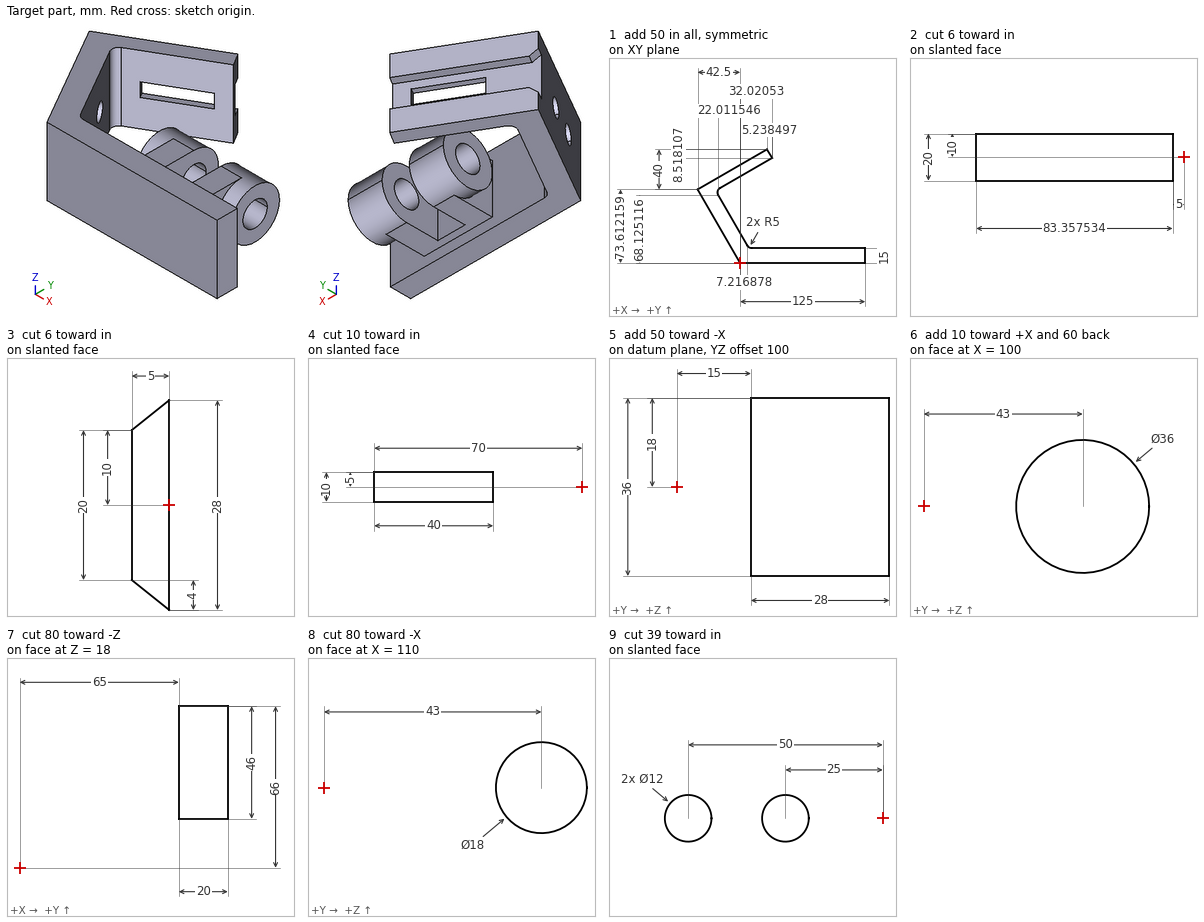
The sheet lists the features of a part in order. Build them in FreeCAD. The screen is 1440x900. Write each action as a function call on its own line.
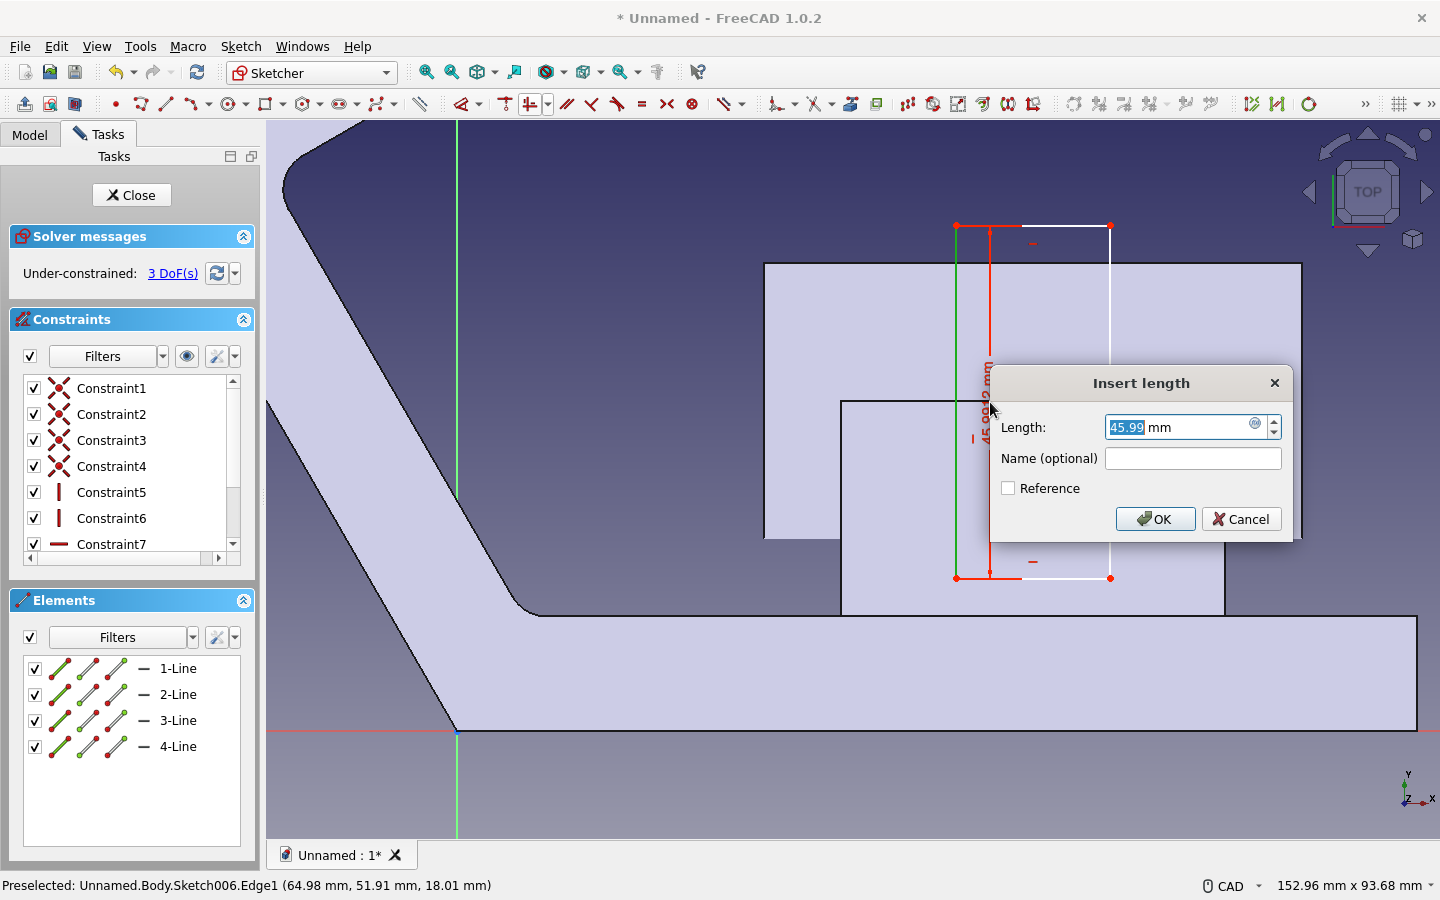
text(46)
key(Return)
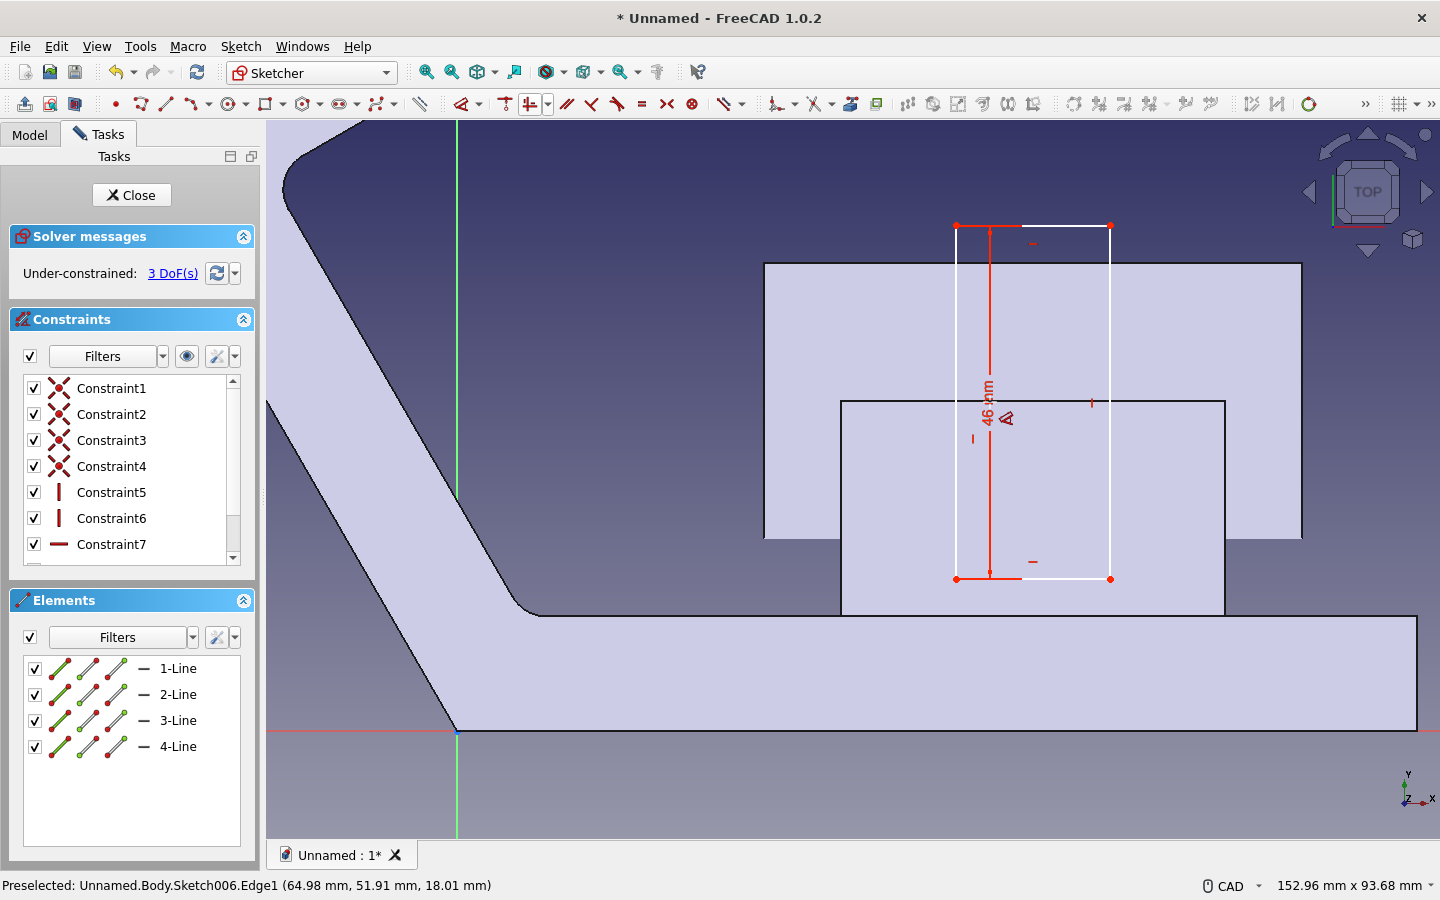
click(1002, 579)
click(1033, 613)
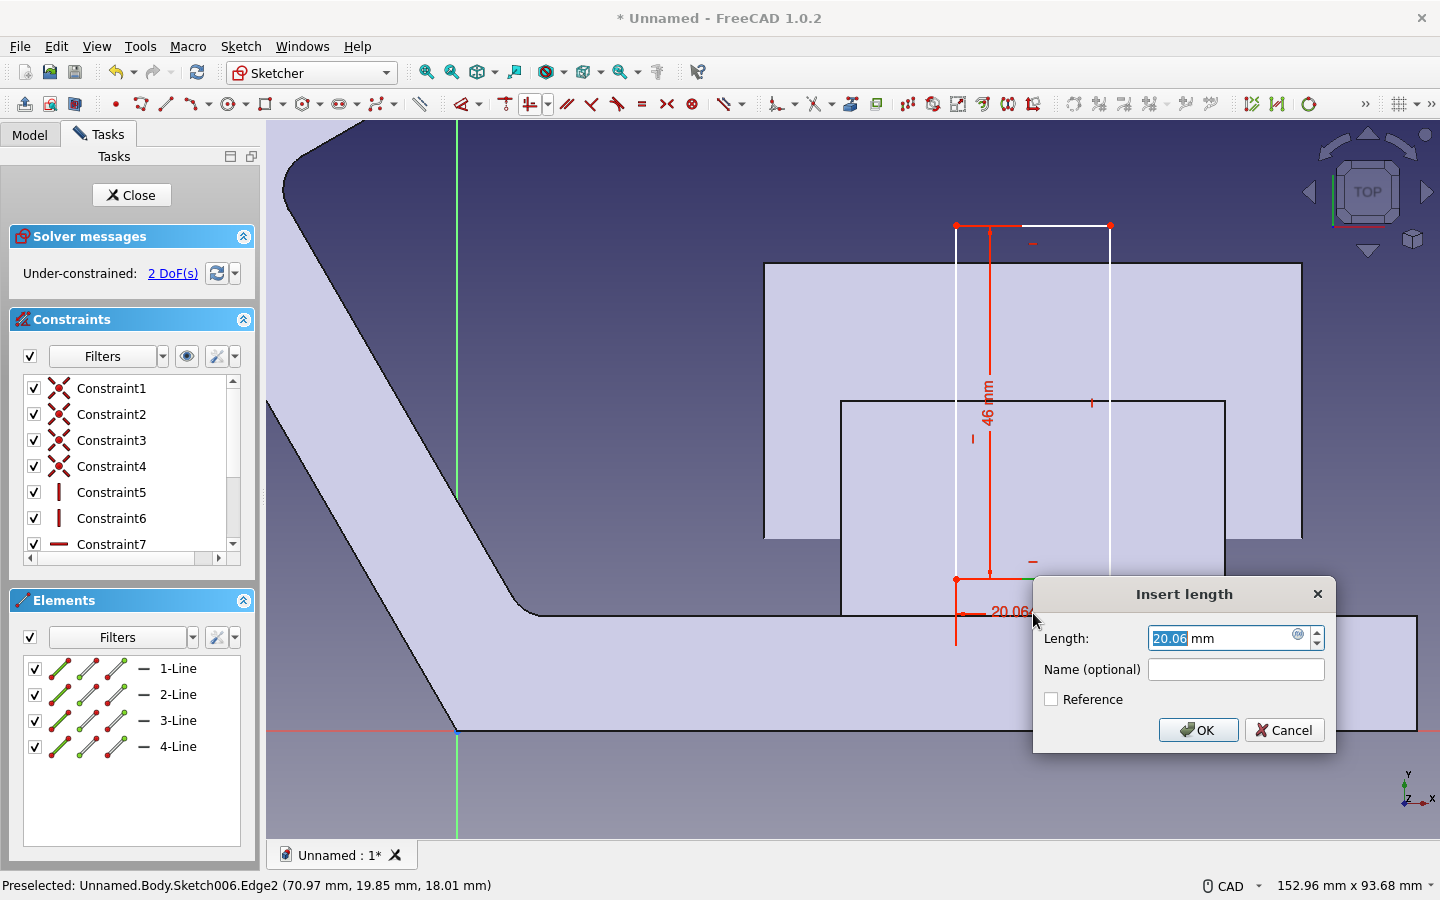
text(20)
key(Return)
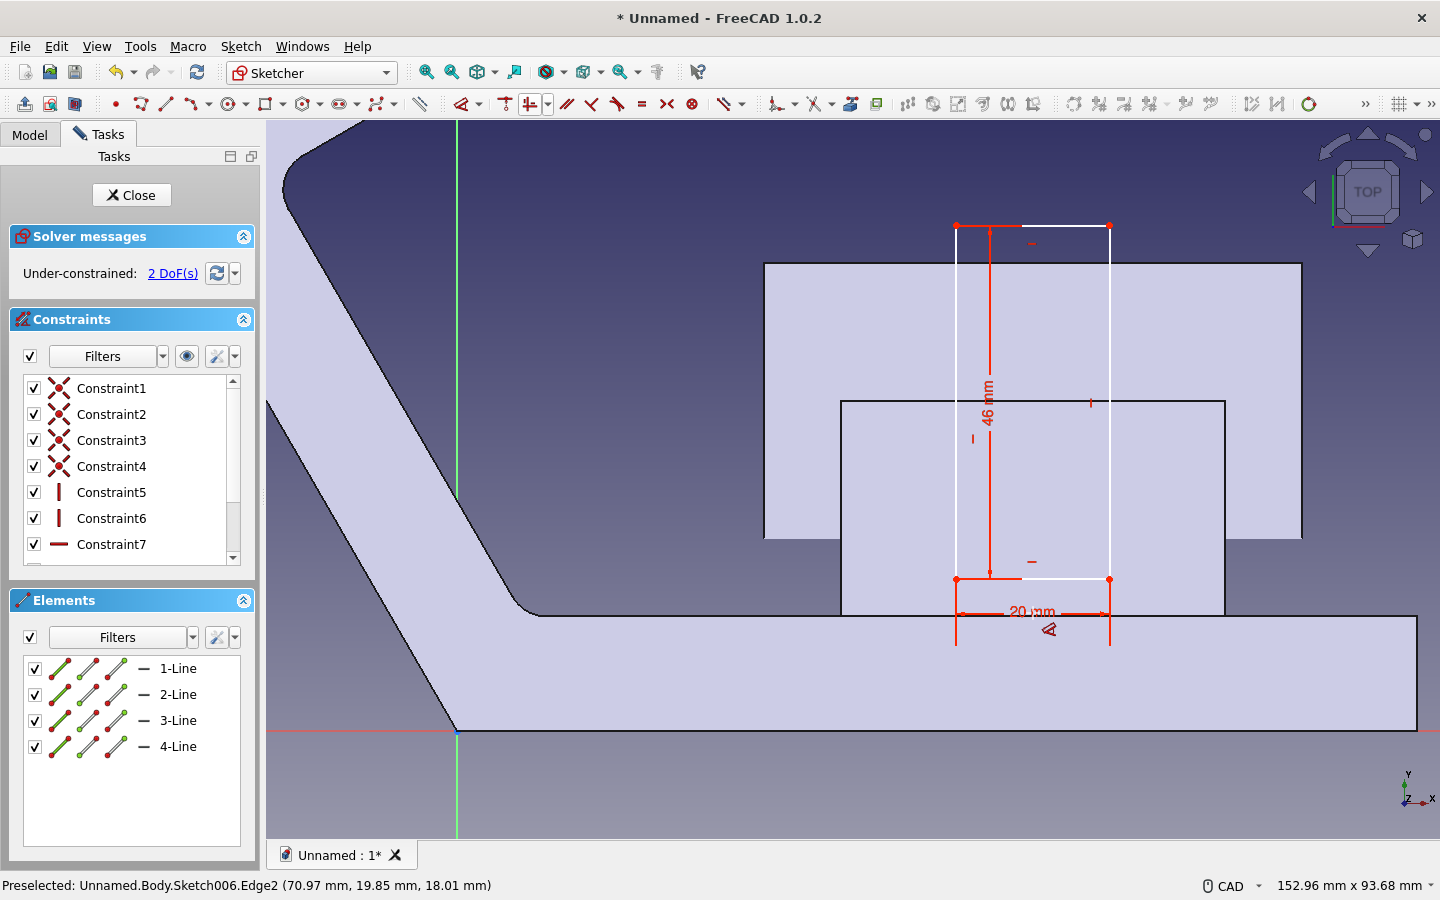
click(956, 226)
click(707, 765)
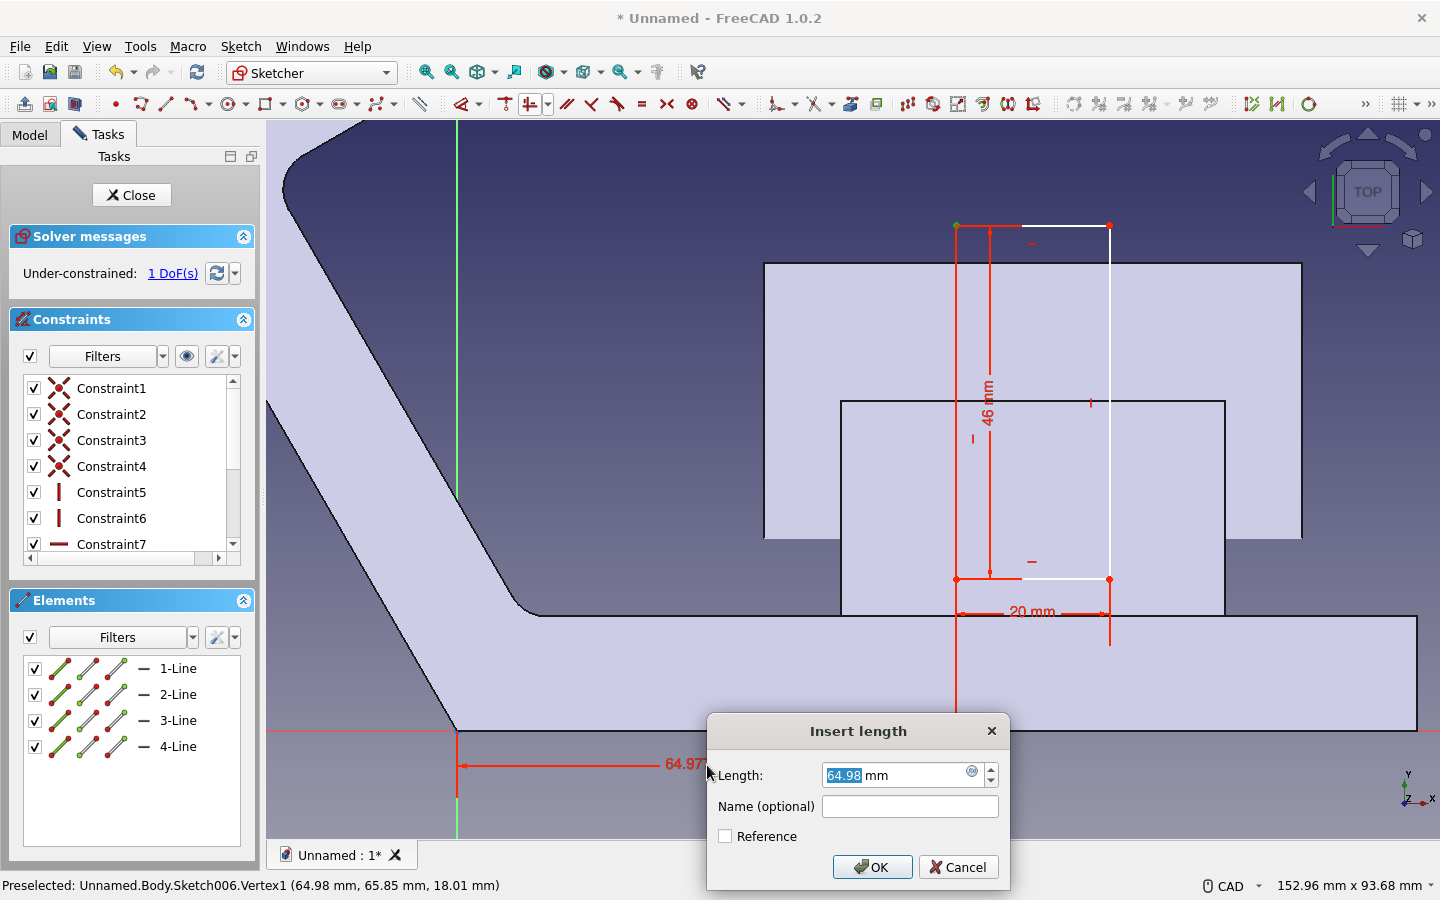
text(65)
key(Return)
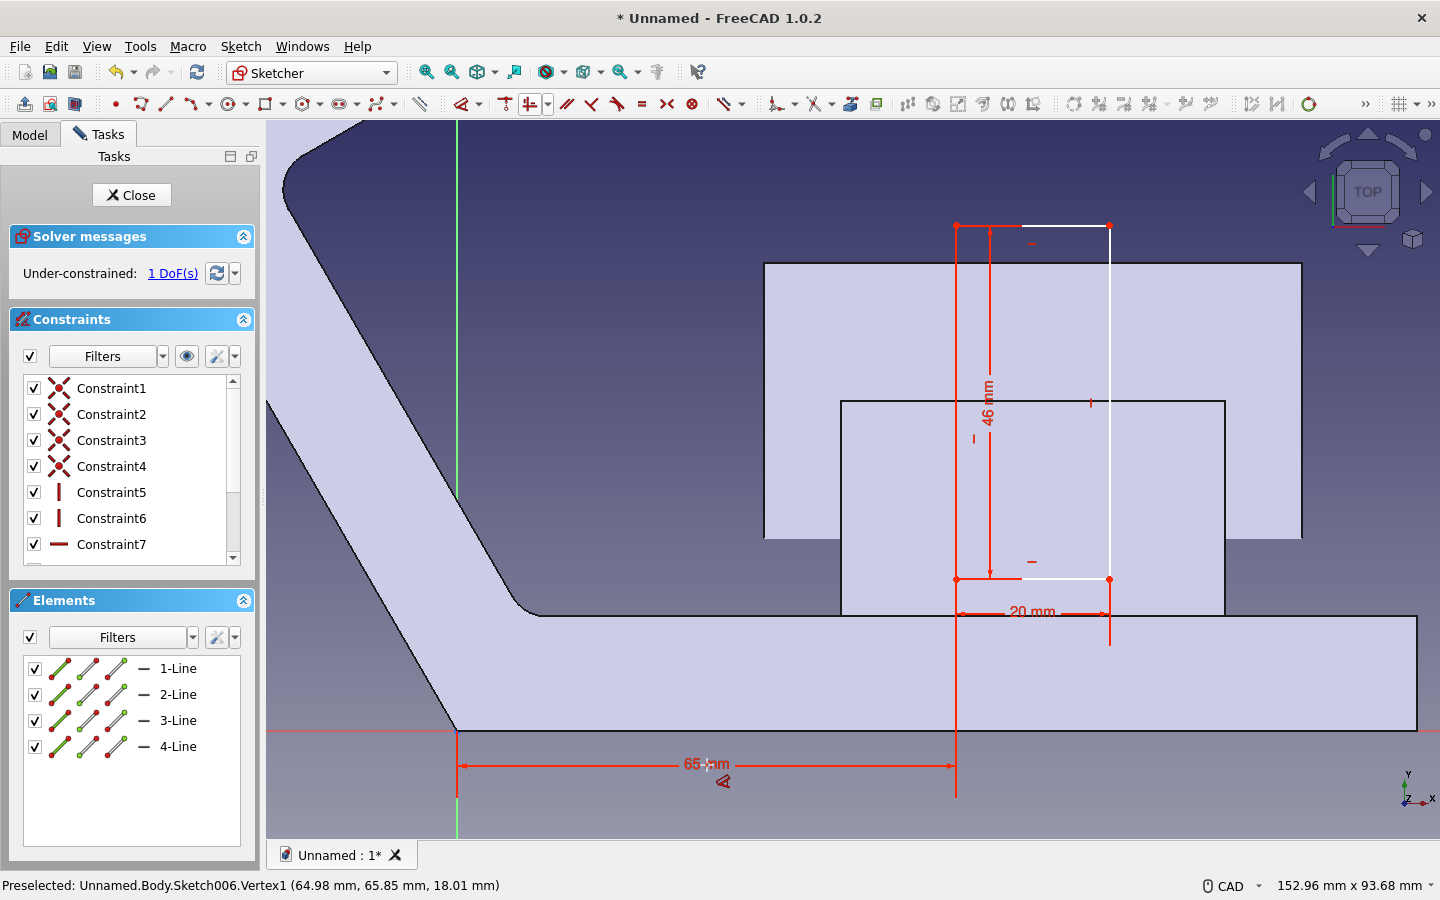
click(956, 226)
click(423, 479)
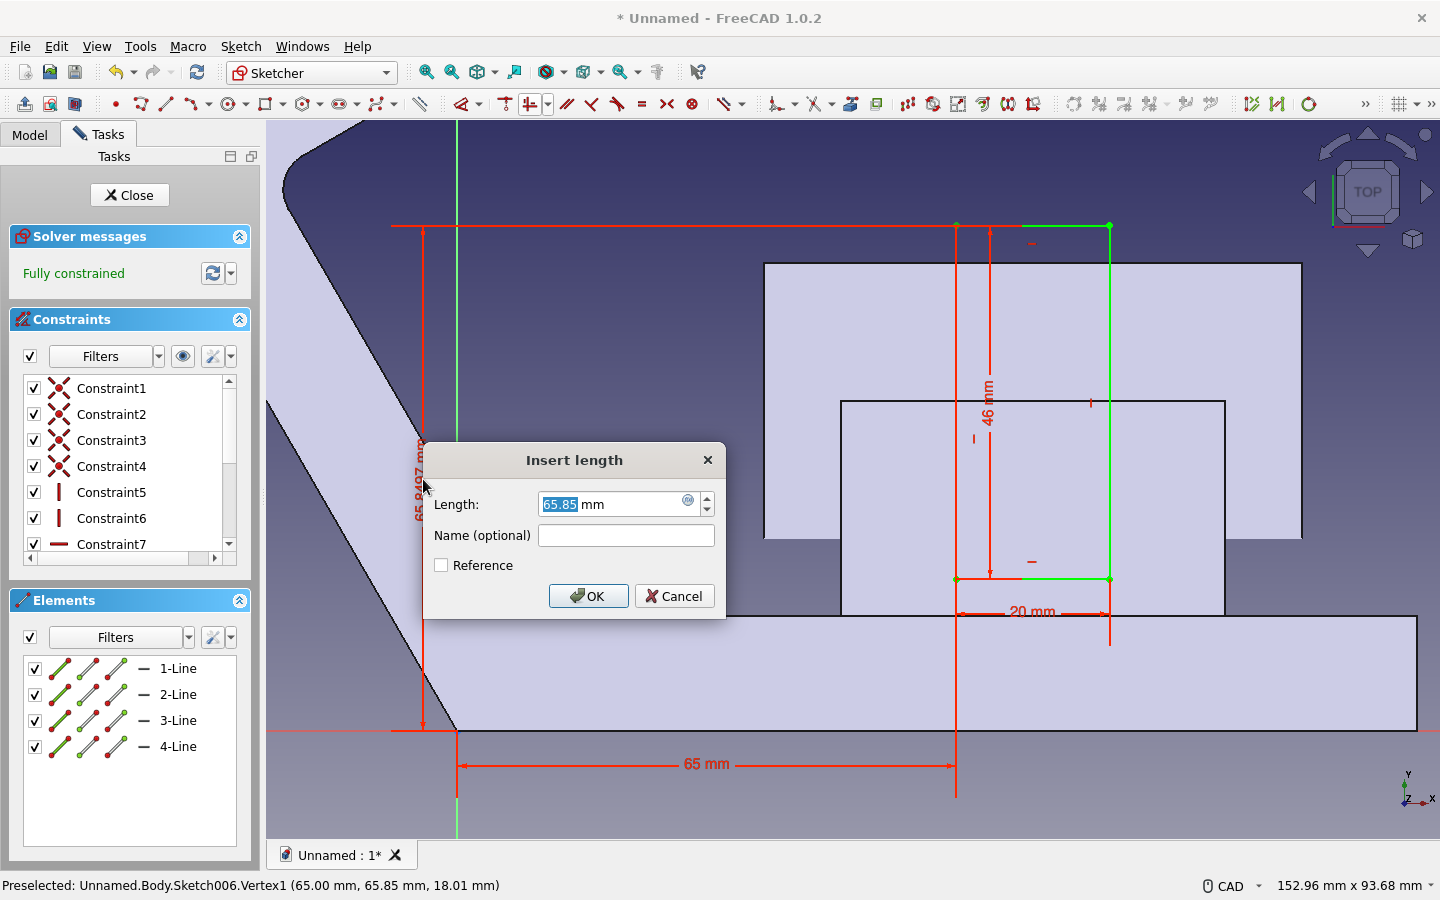
text(66)
key(Return)
key(Escape)